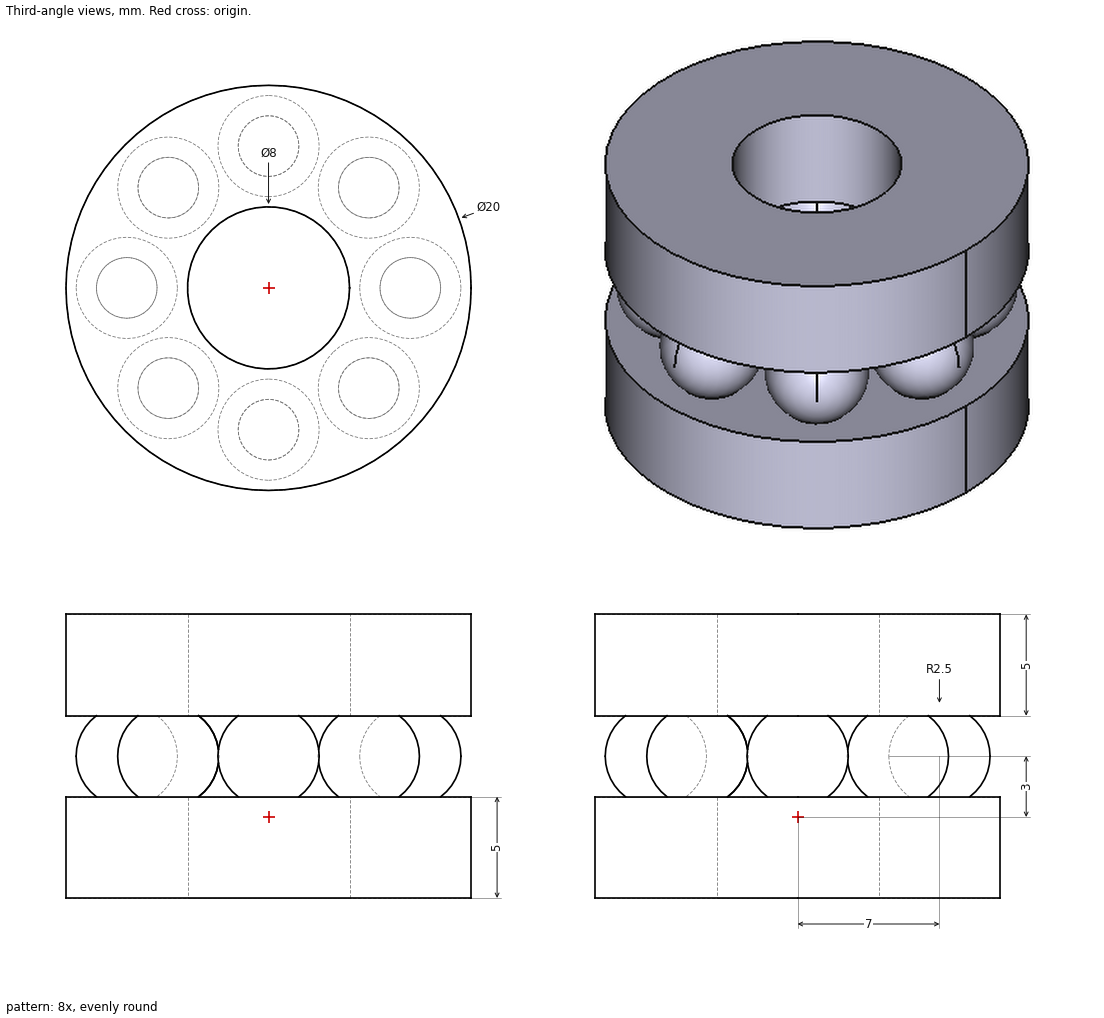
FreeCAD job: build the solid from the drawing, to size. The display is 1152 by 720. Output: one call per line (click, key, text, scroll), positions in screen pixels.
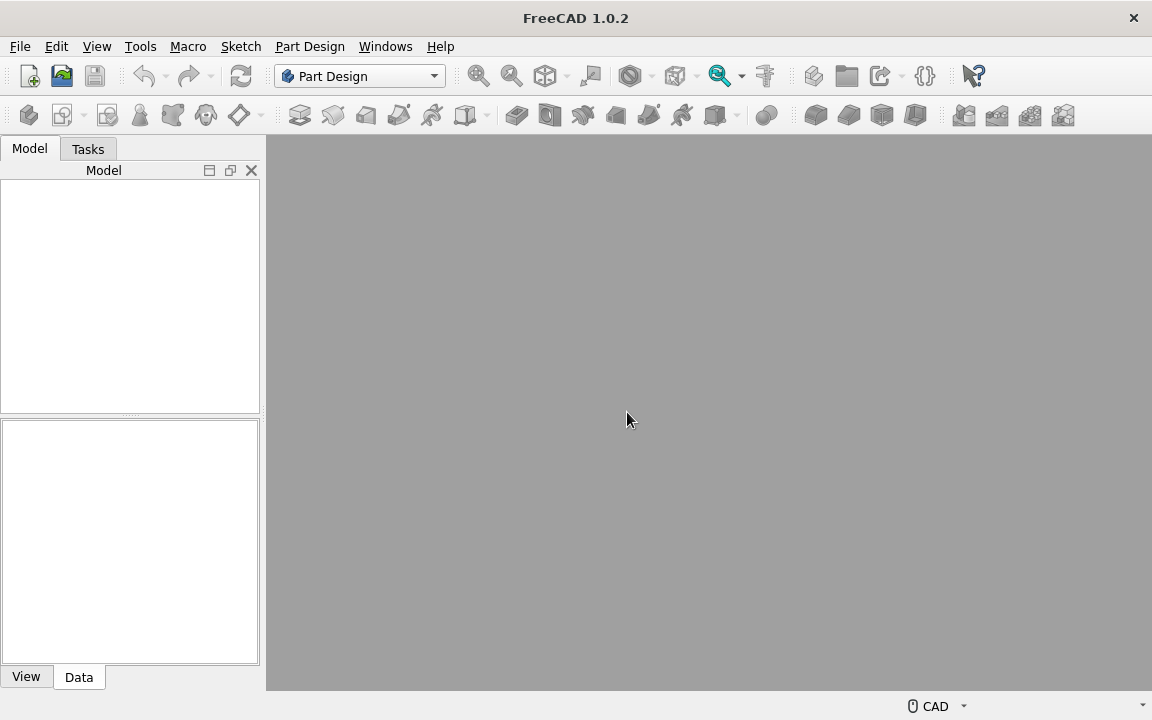
click(29, 76)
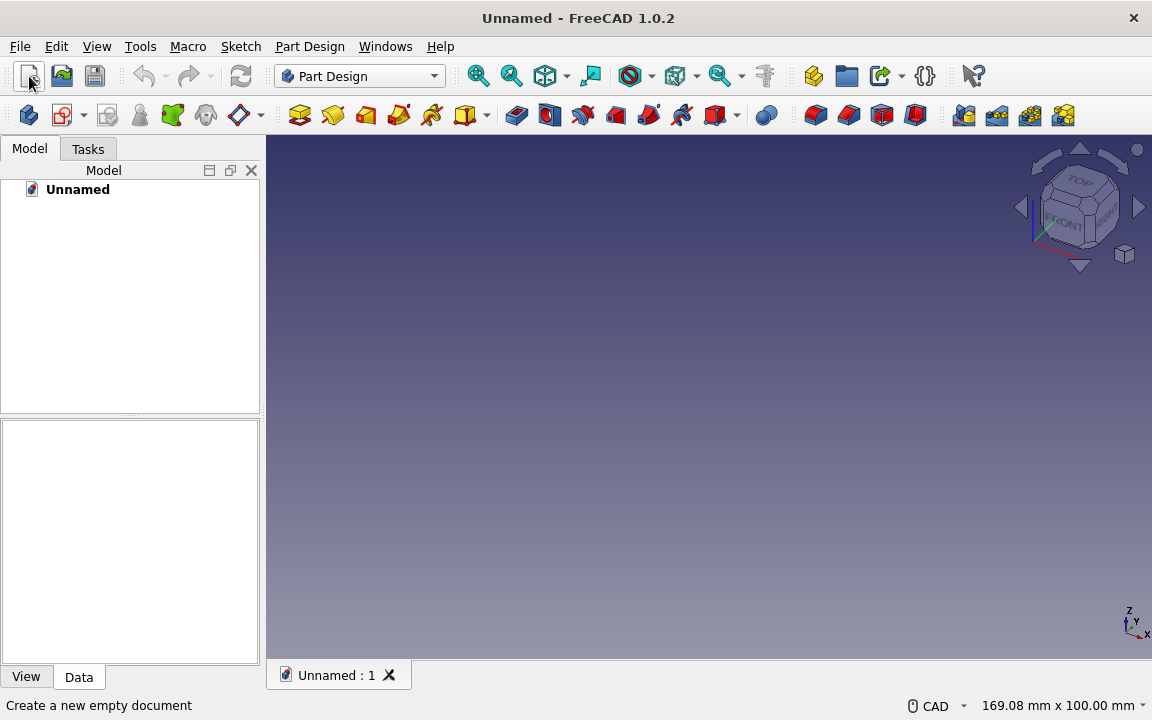
click(29, 116)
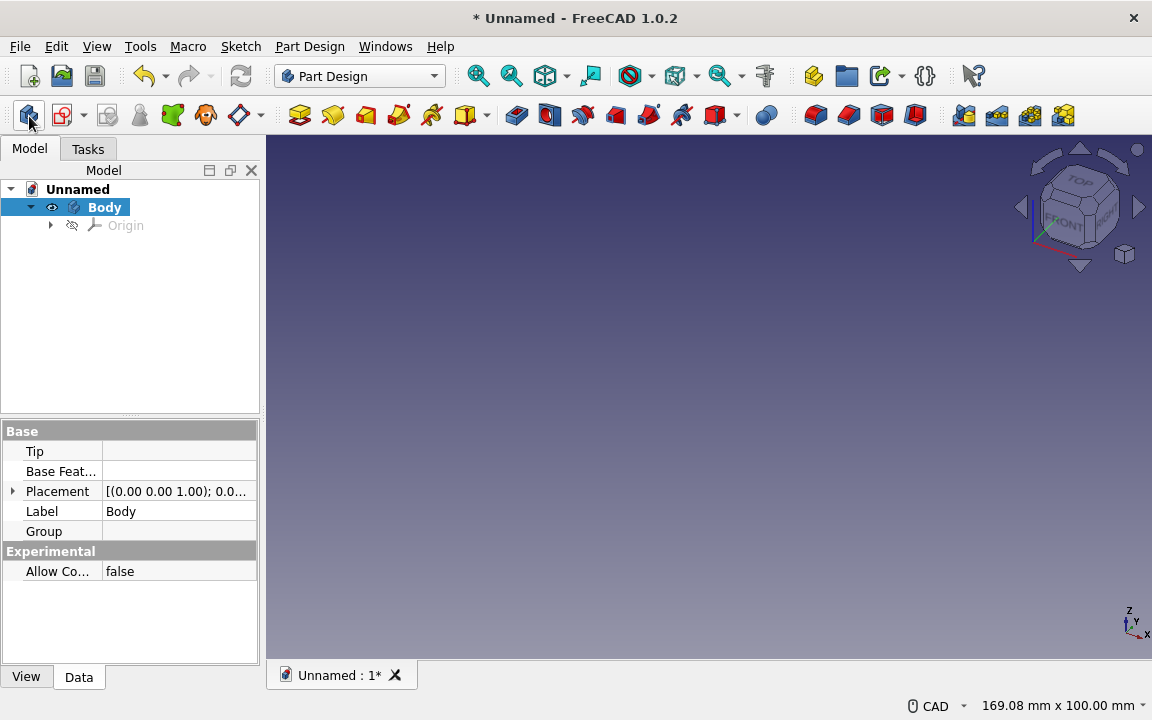
click(51, 225)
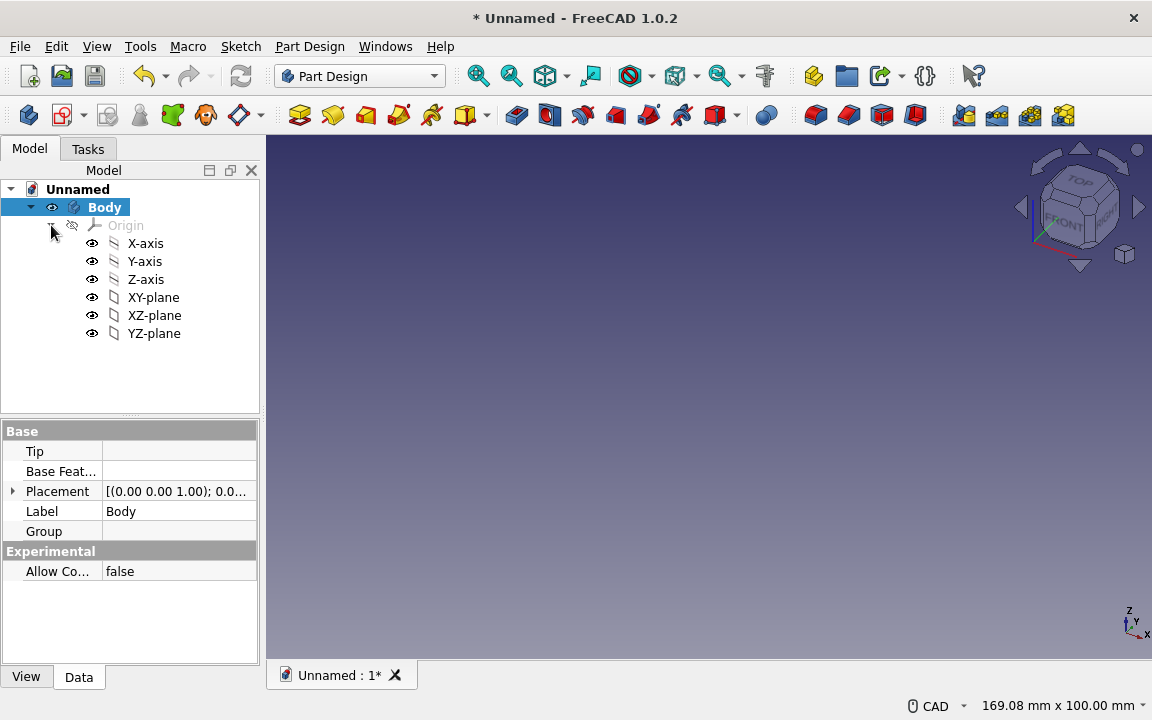
click(137, 297)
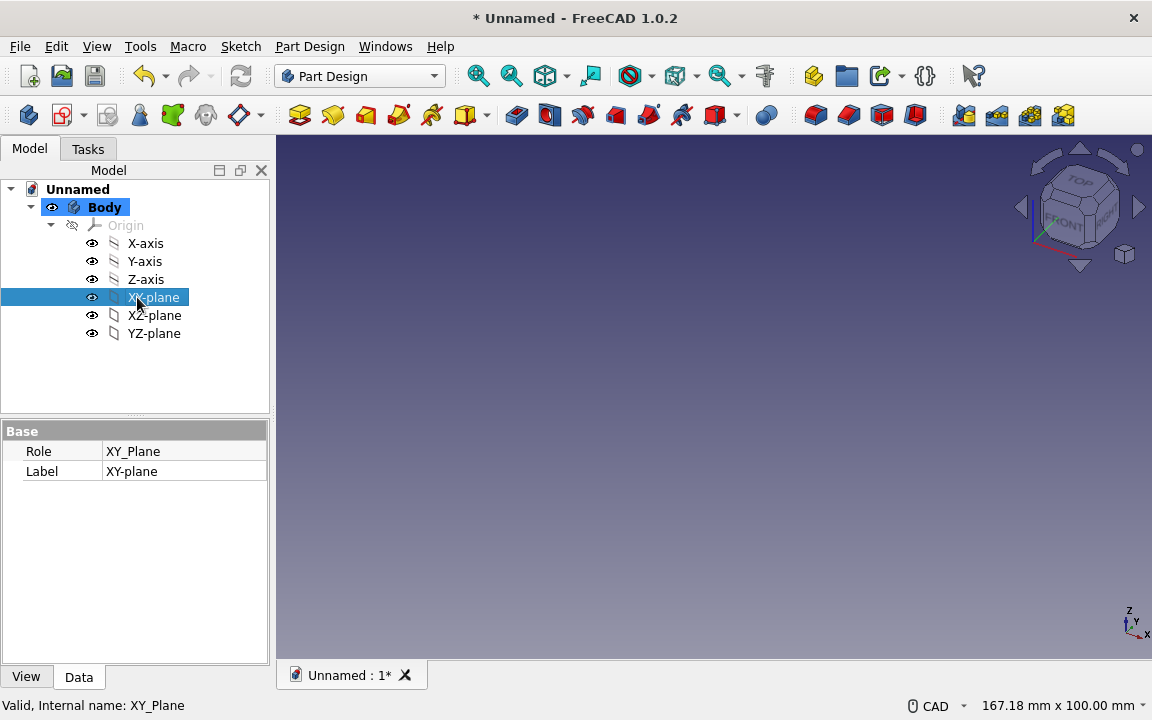
click(238, 116)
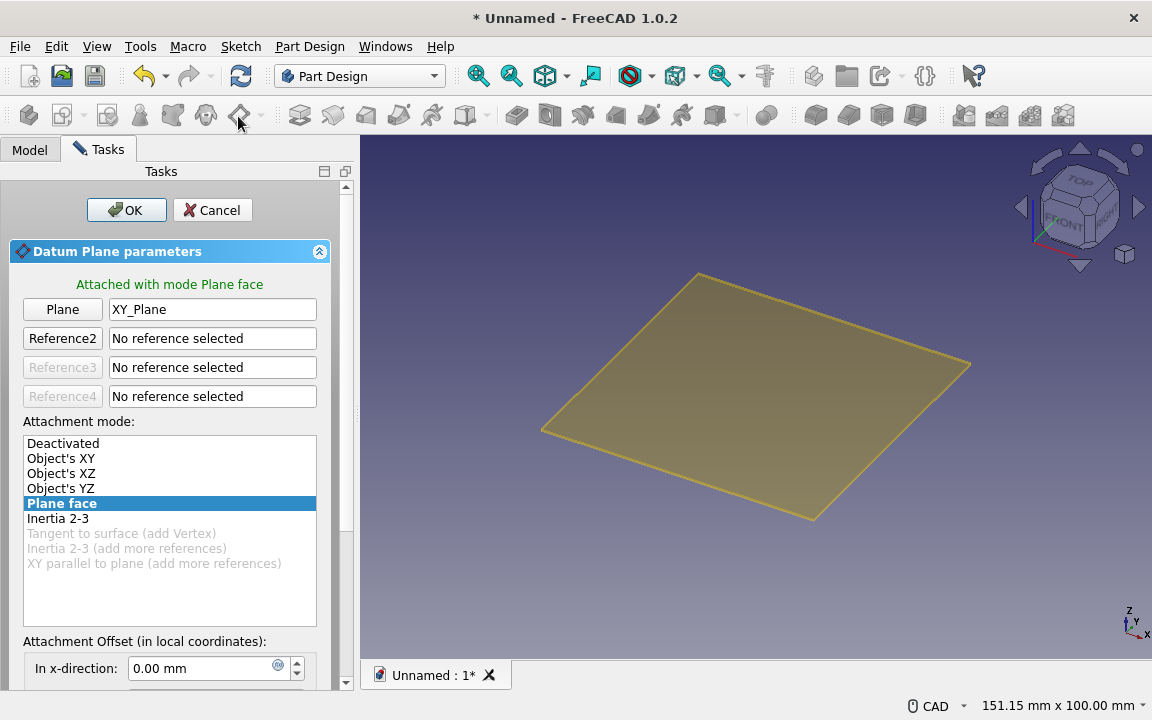
scroll(346, 436, down, 2)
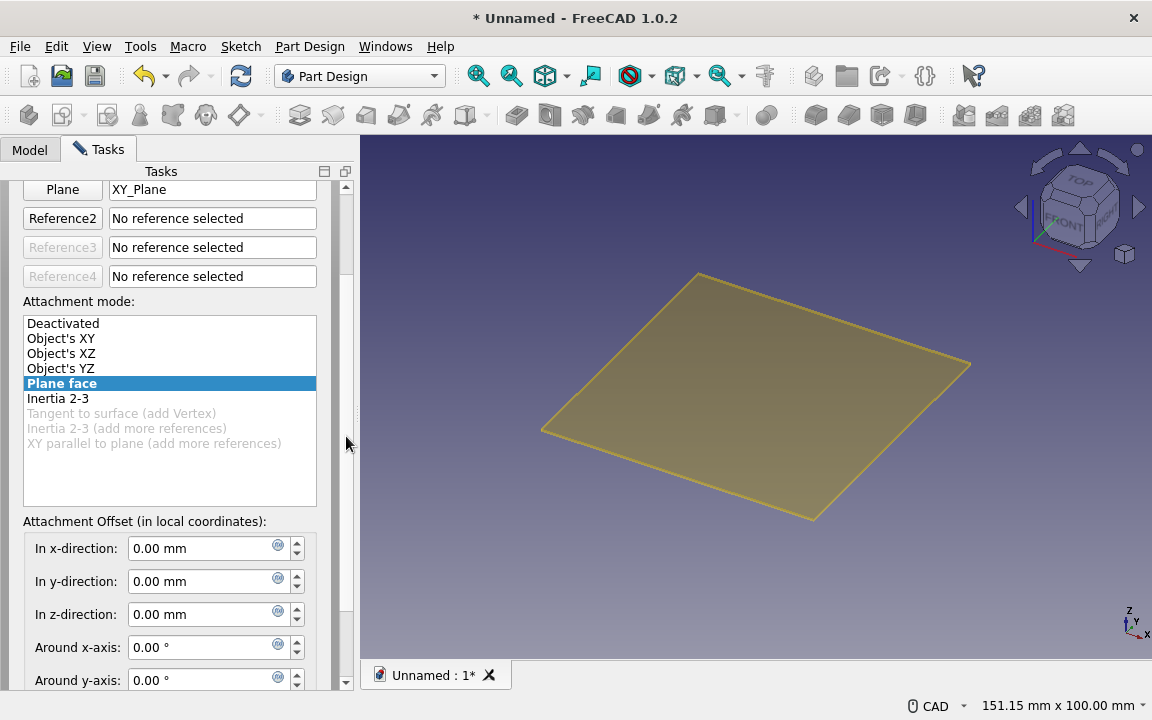
triple_click(210, 614)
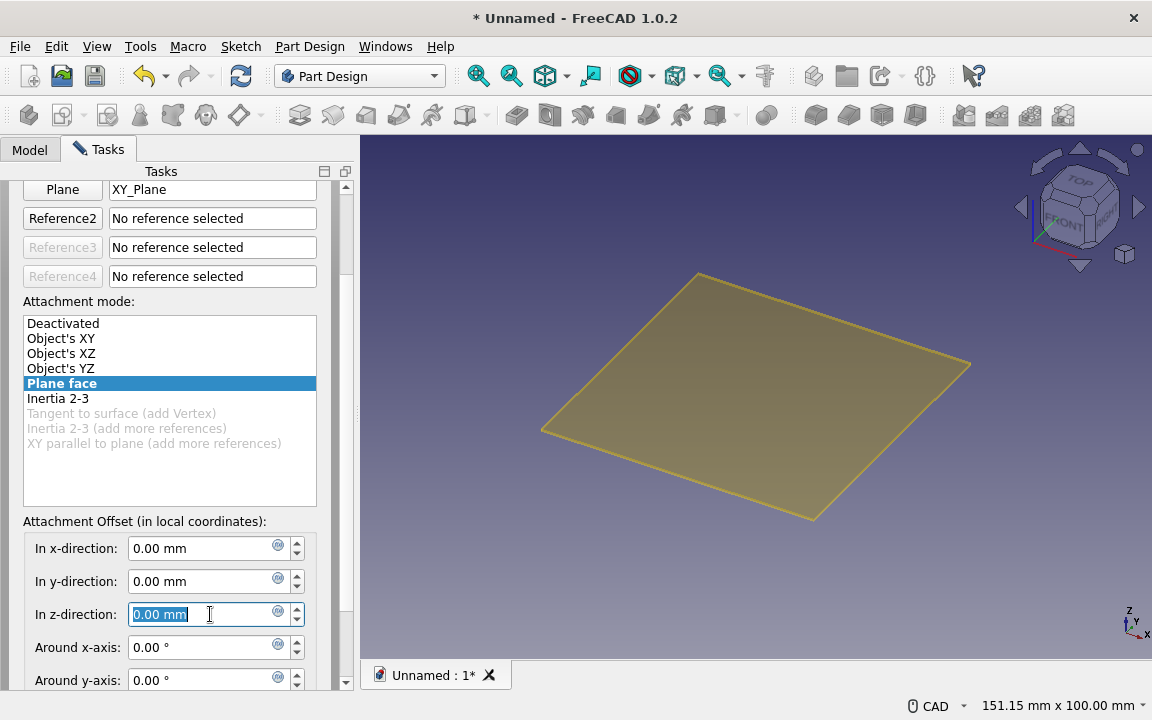
text(5)
key(Tab)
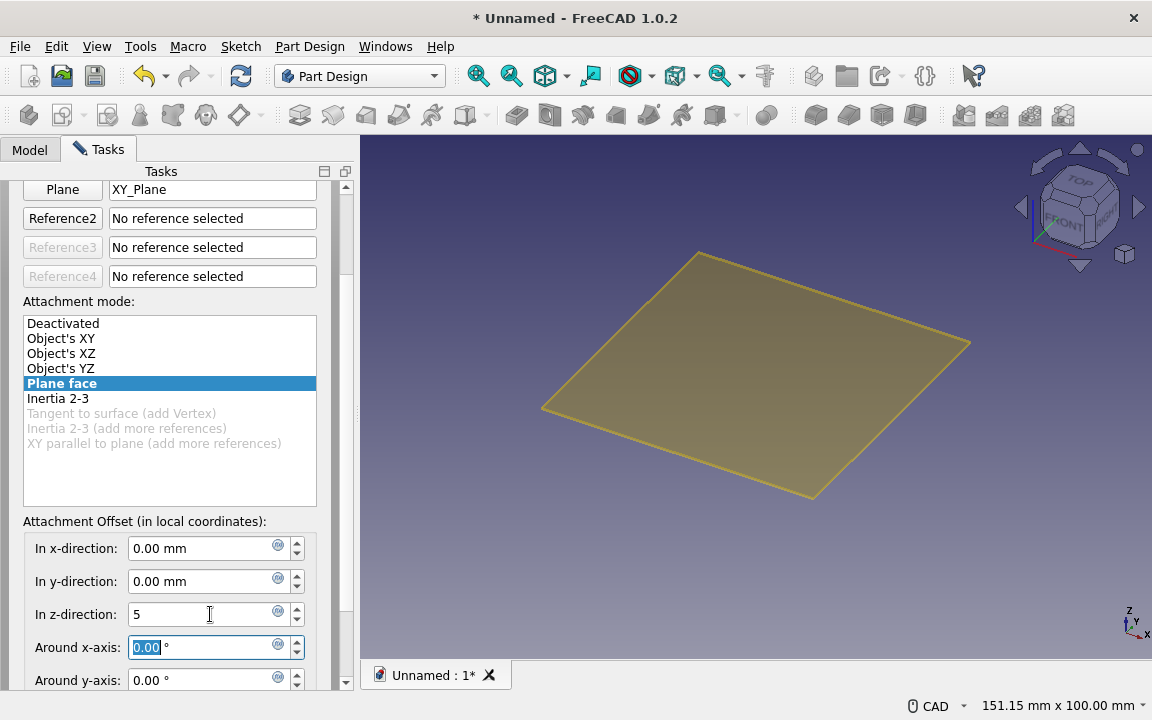
scroll(346, 436, up, 3)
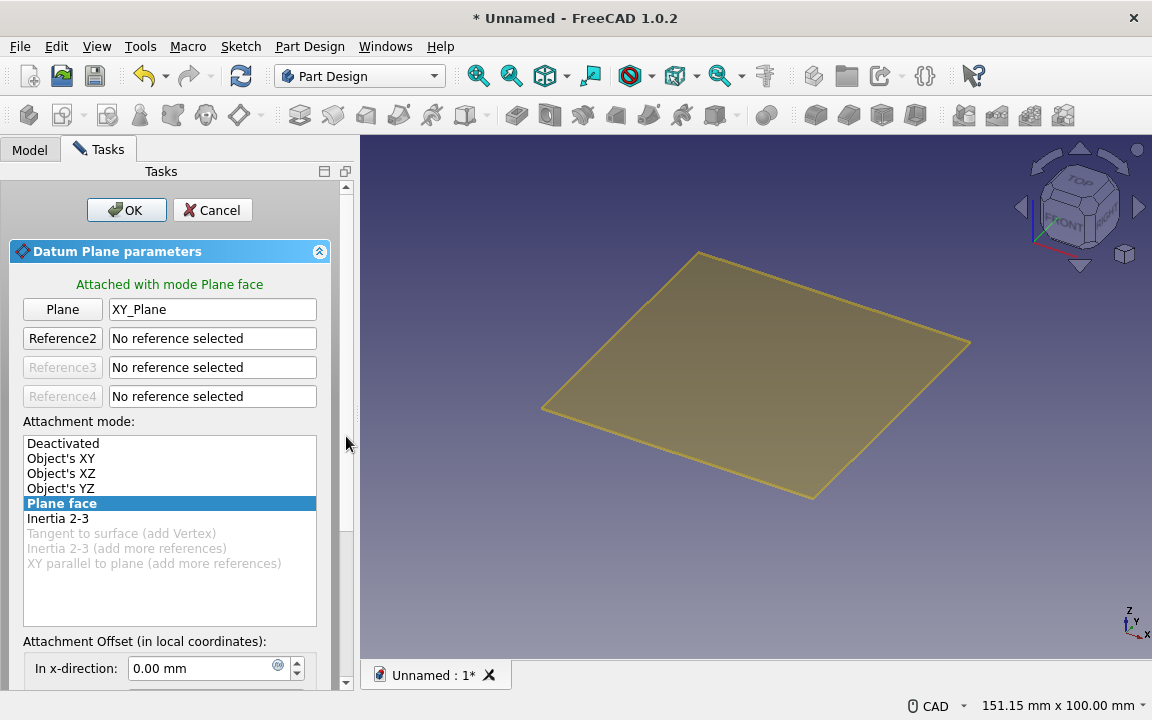
click(127, 210)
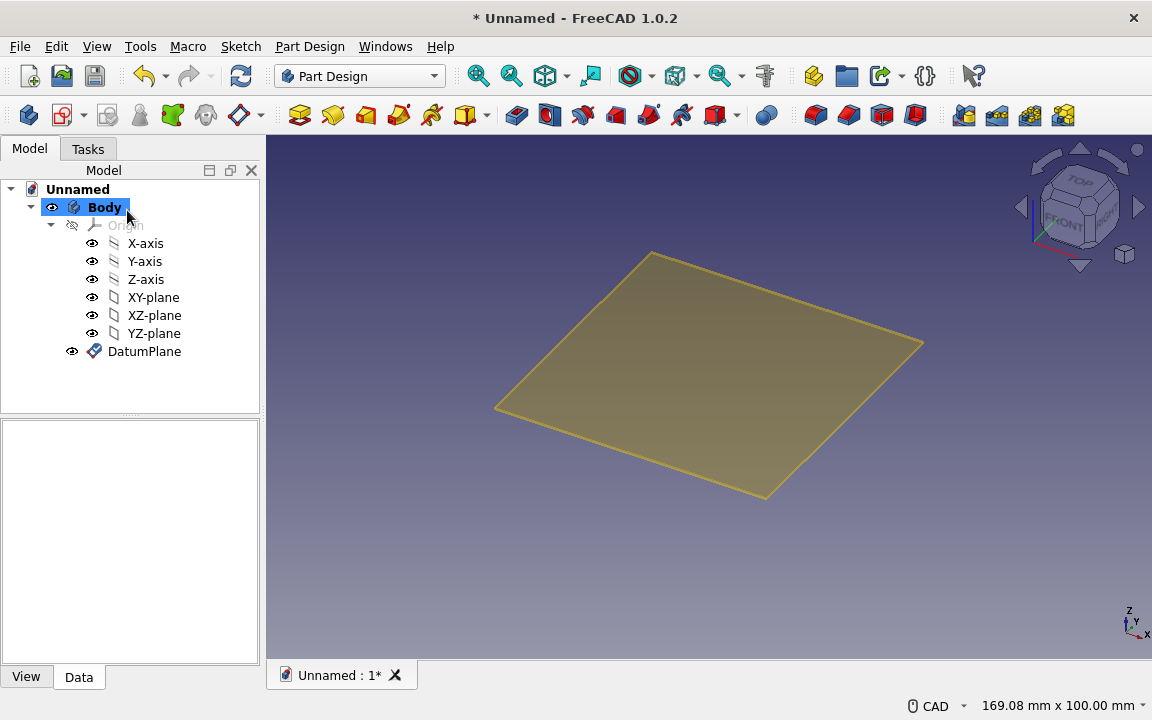
click(117, 351)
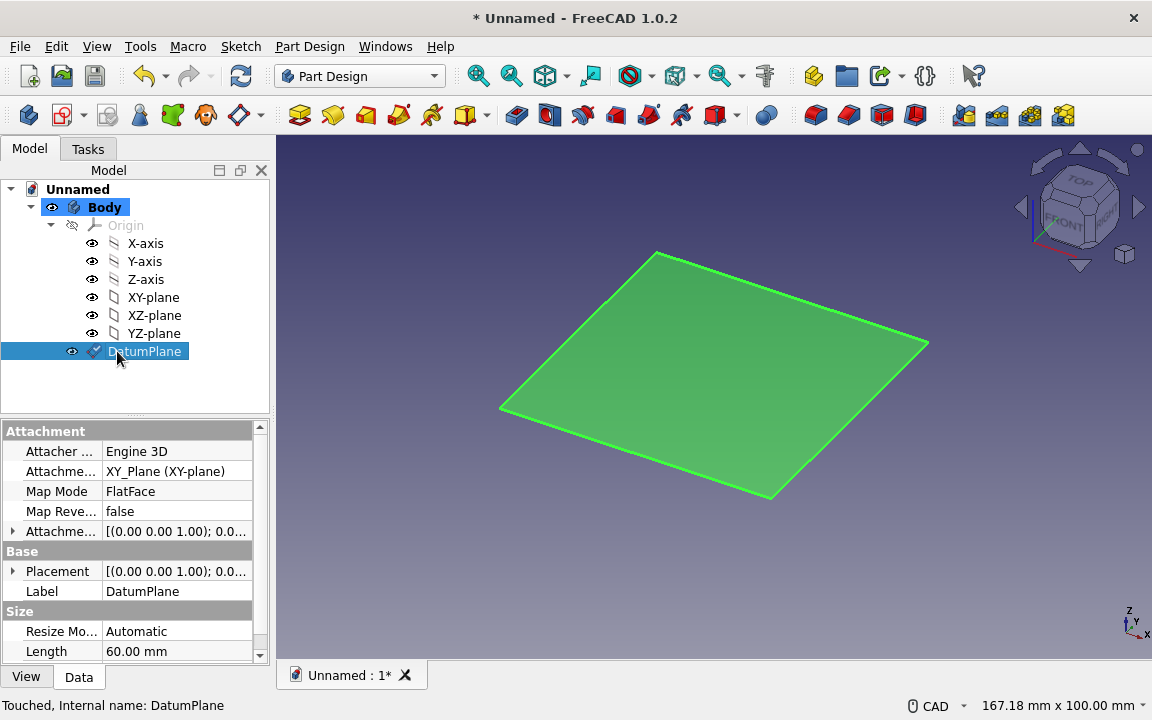
click(62, 116)